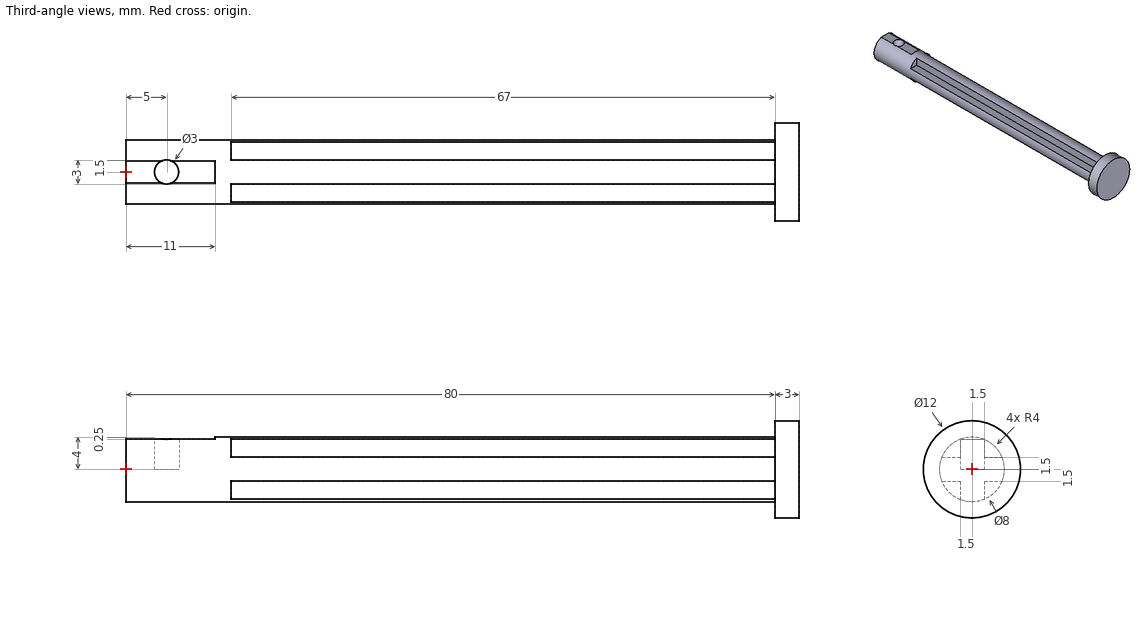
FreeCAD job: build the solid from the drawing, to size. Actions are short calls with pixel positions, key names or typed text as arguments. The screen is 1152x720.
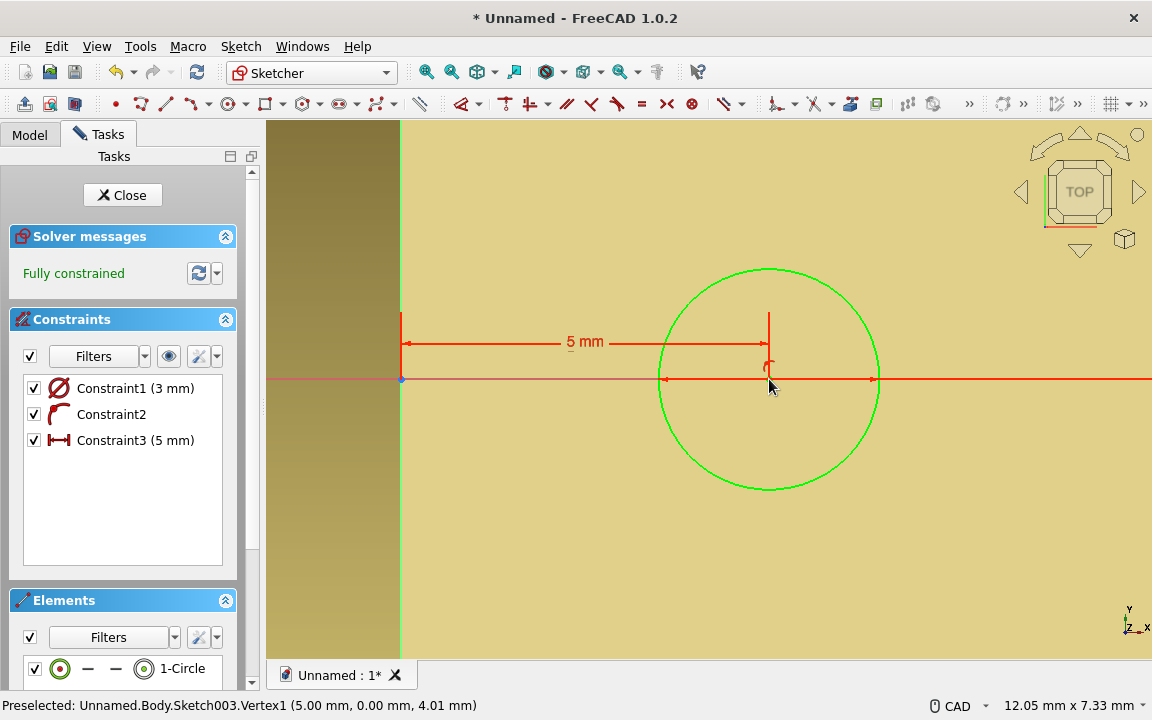
click(123, 195)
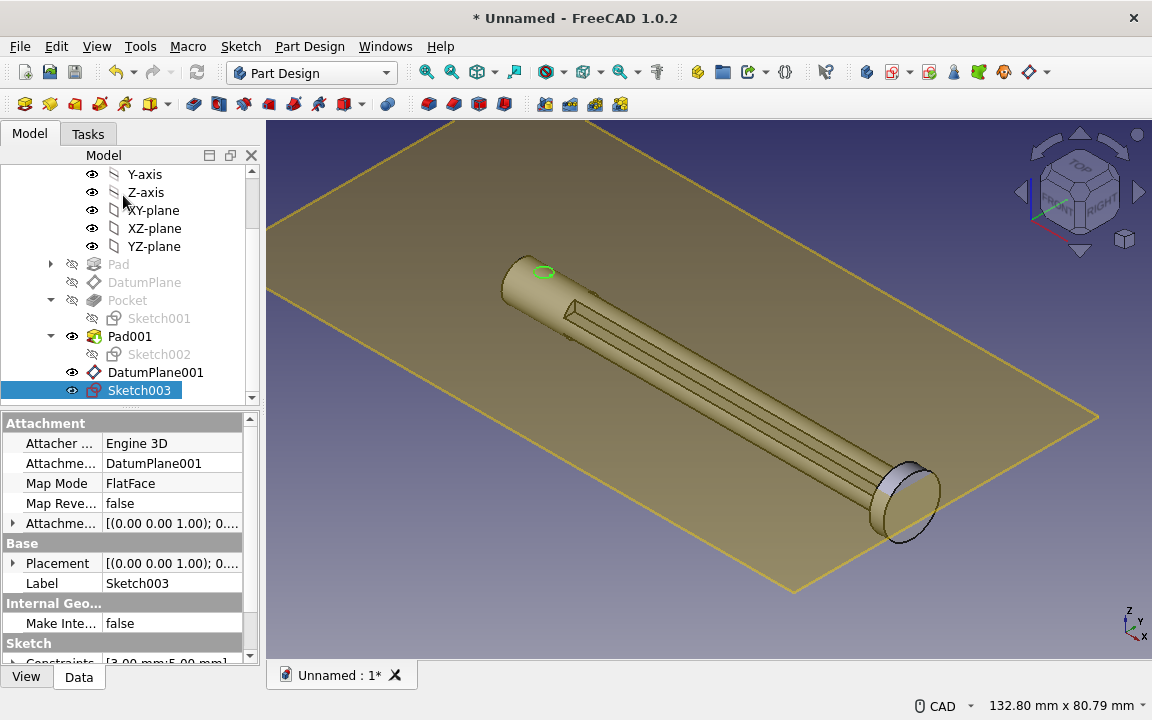
click(194, 104)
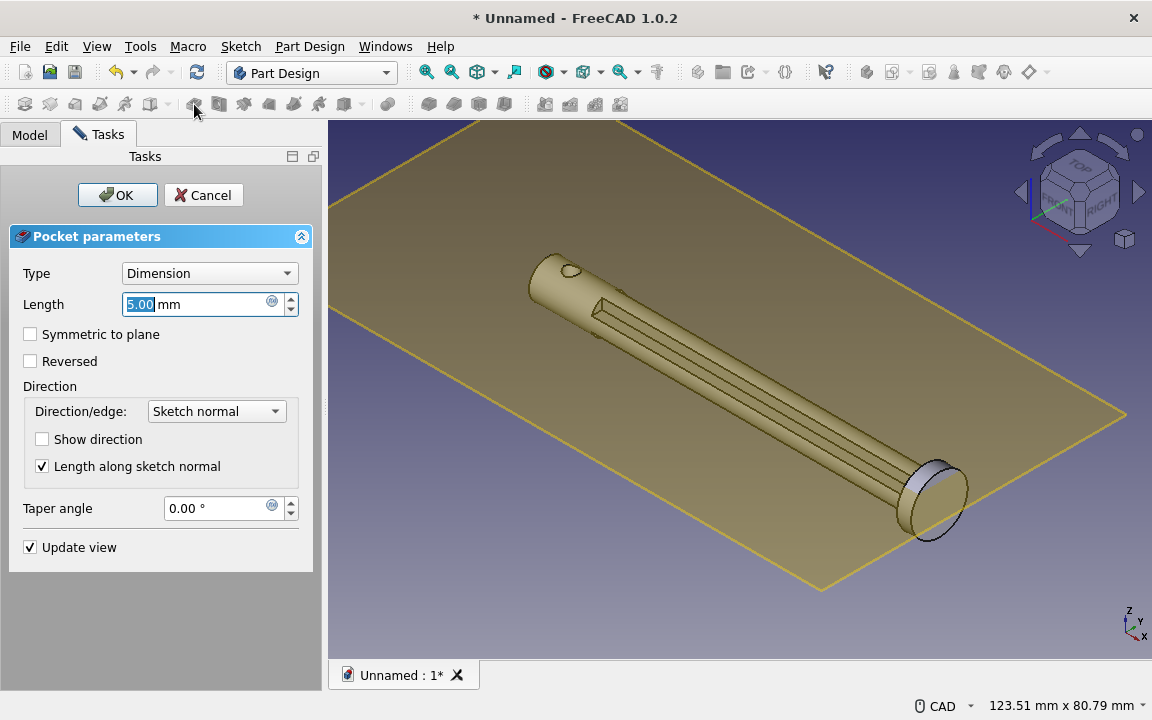
text(4)
key(Tab)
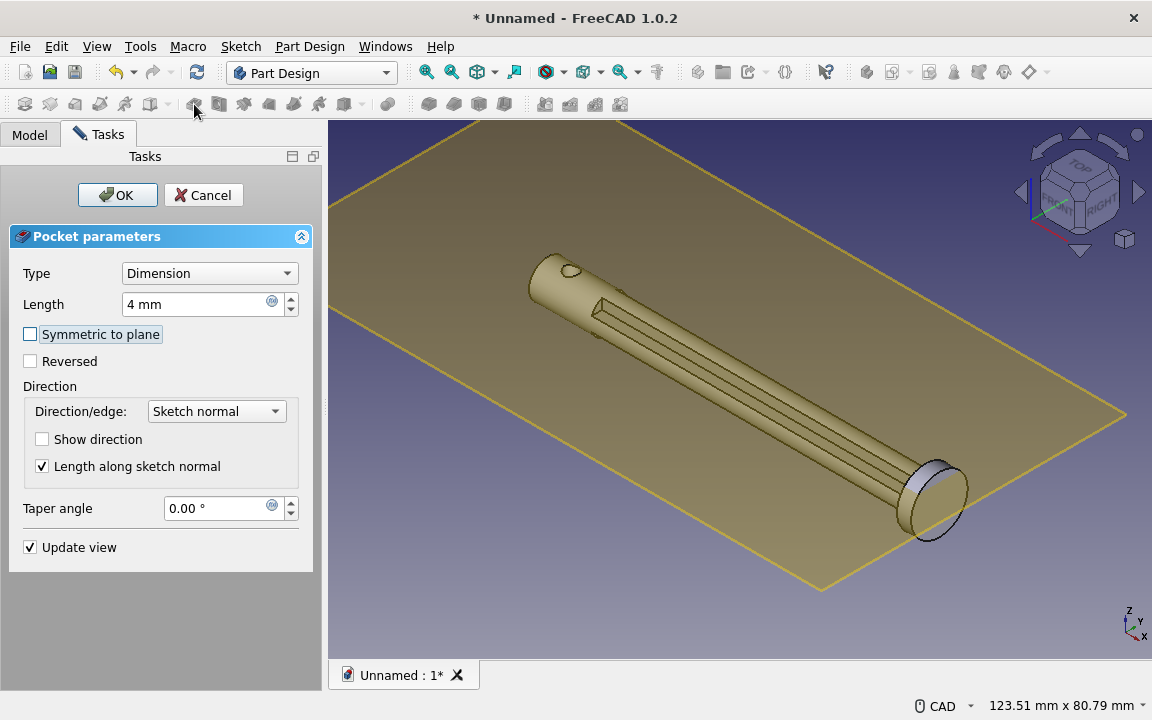
click(118, 195)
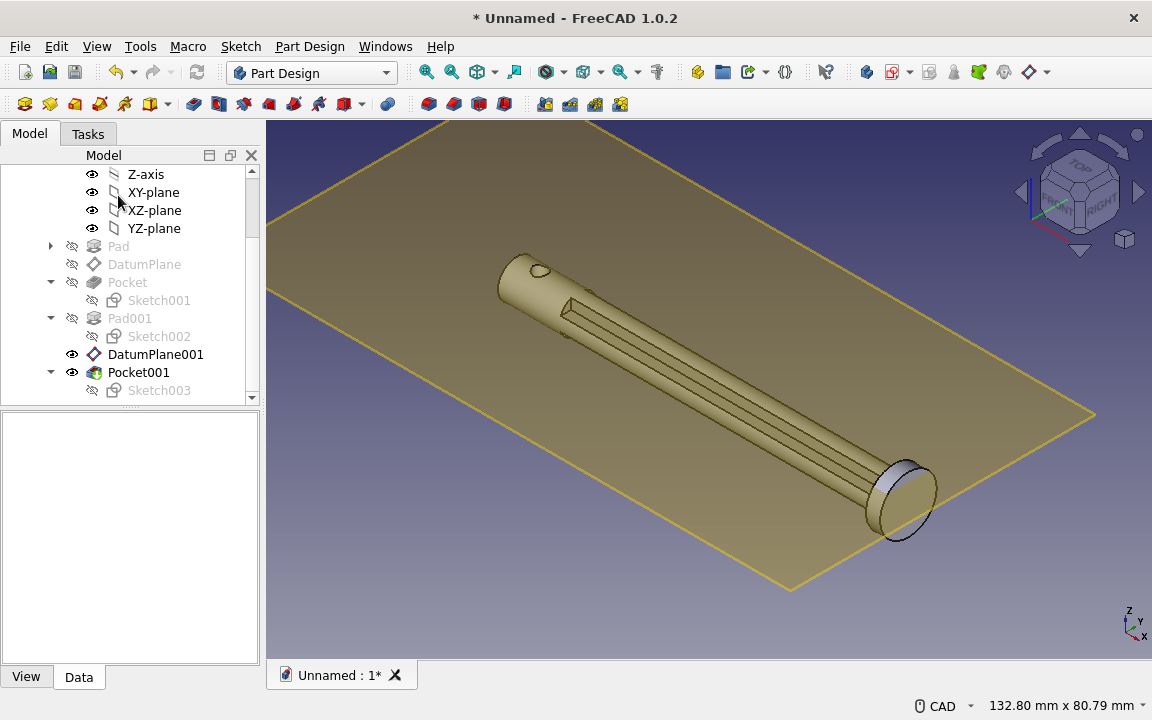
click(117, 354)
key(space)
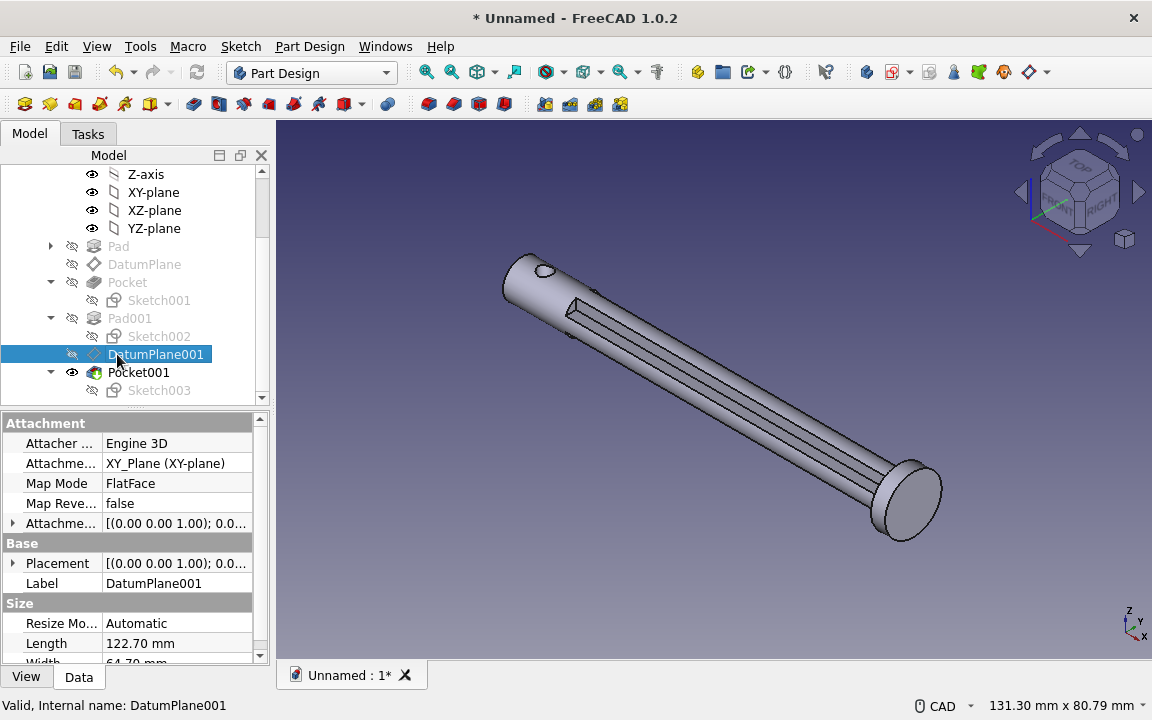
scroll(161, 278, down, 3)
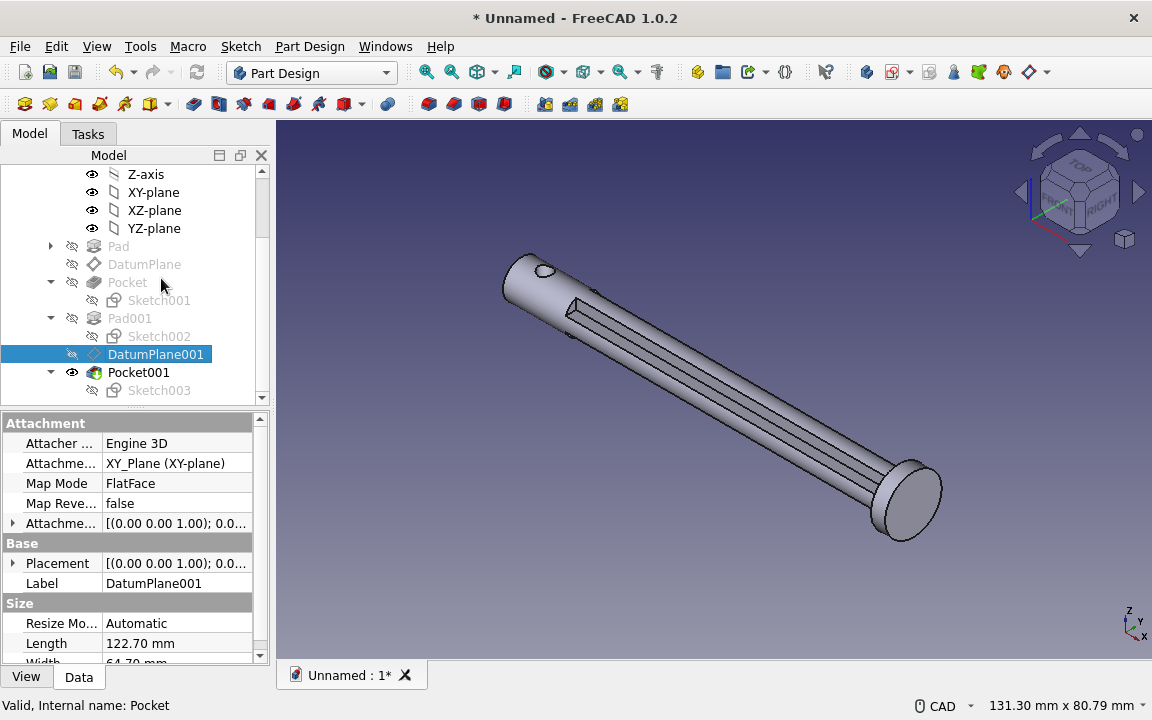
scroll(161, 278, up, 15)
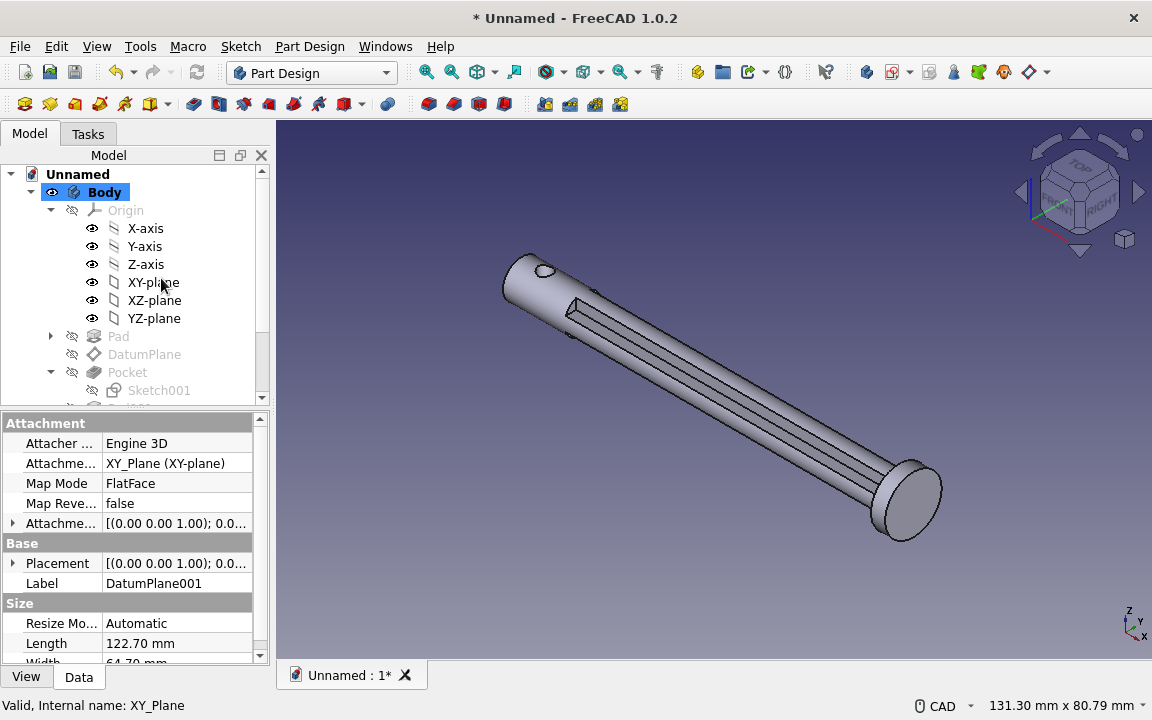
click(137, 282)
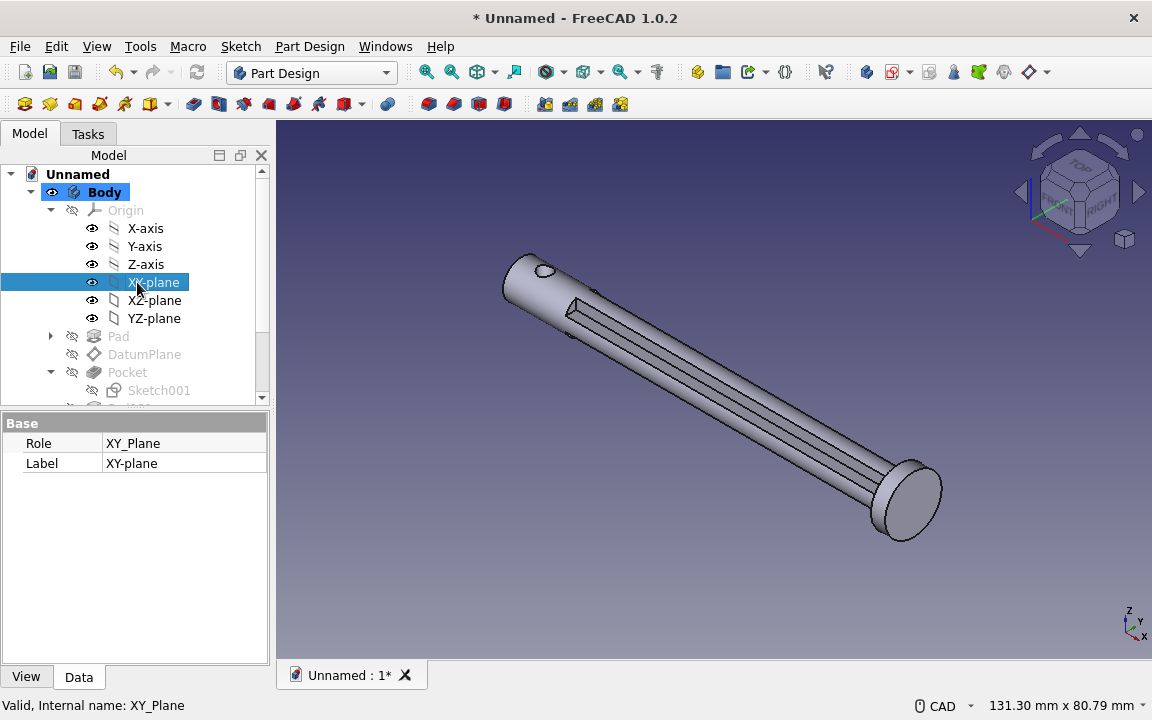
click(1028, 72)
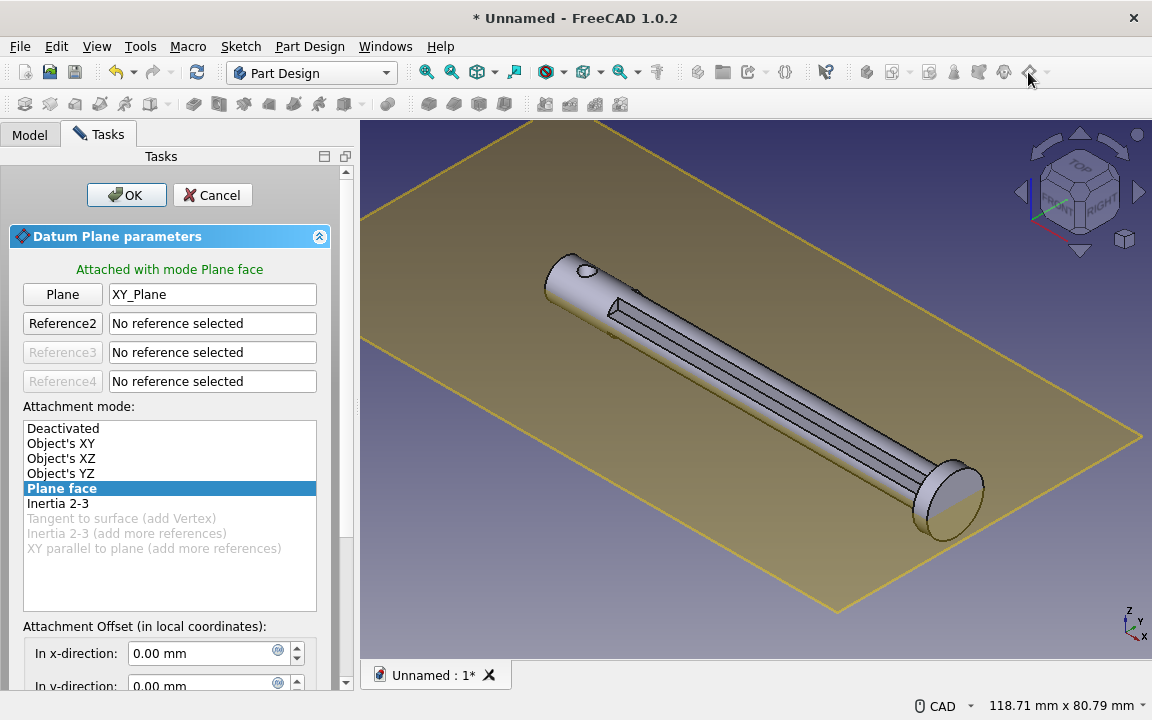
scroll(346, 428, down, 2)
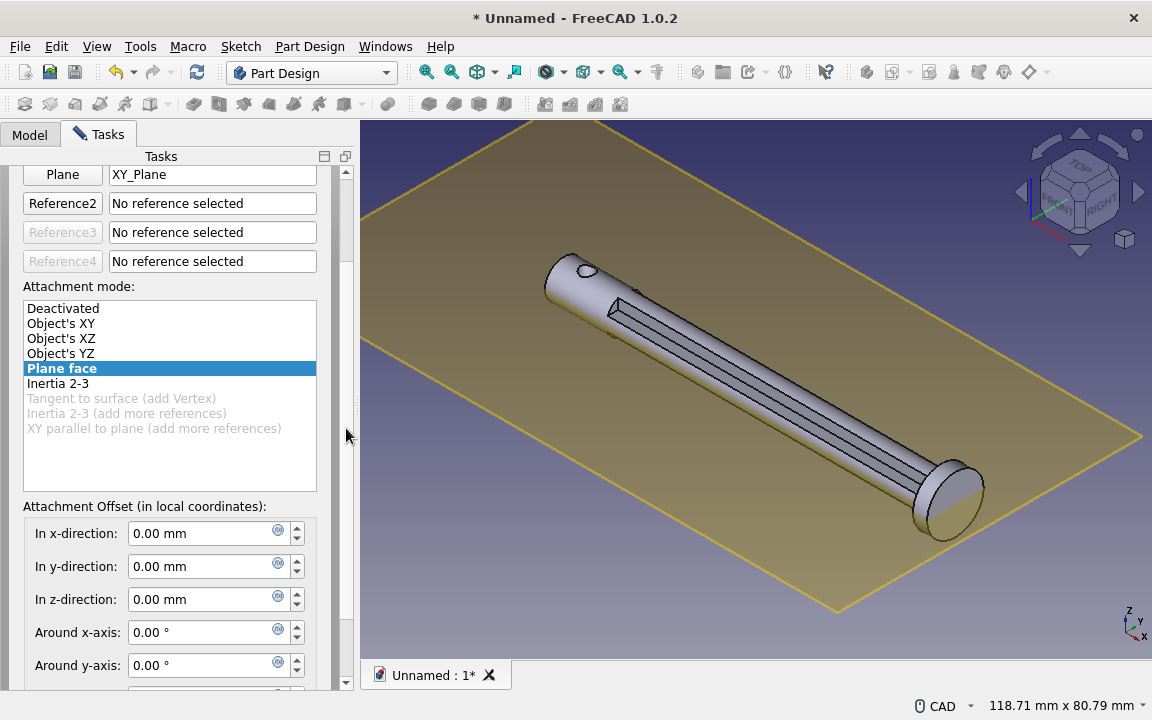
triple_click(210, 600)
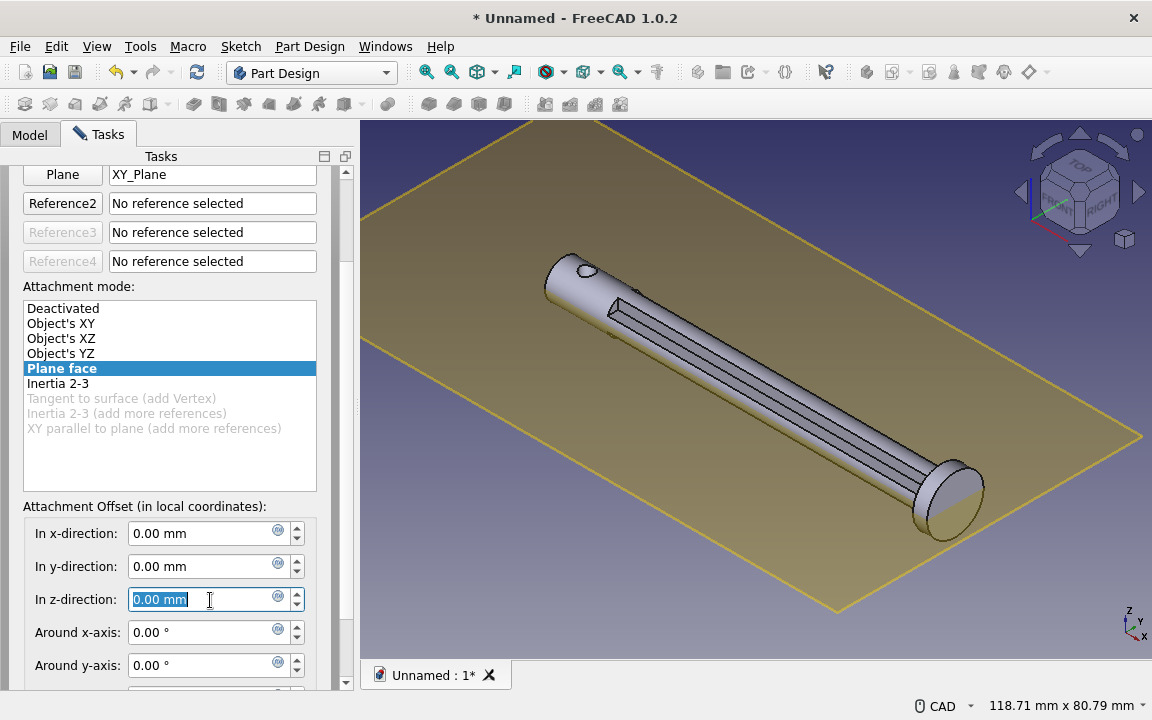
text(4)
key(Tab)